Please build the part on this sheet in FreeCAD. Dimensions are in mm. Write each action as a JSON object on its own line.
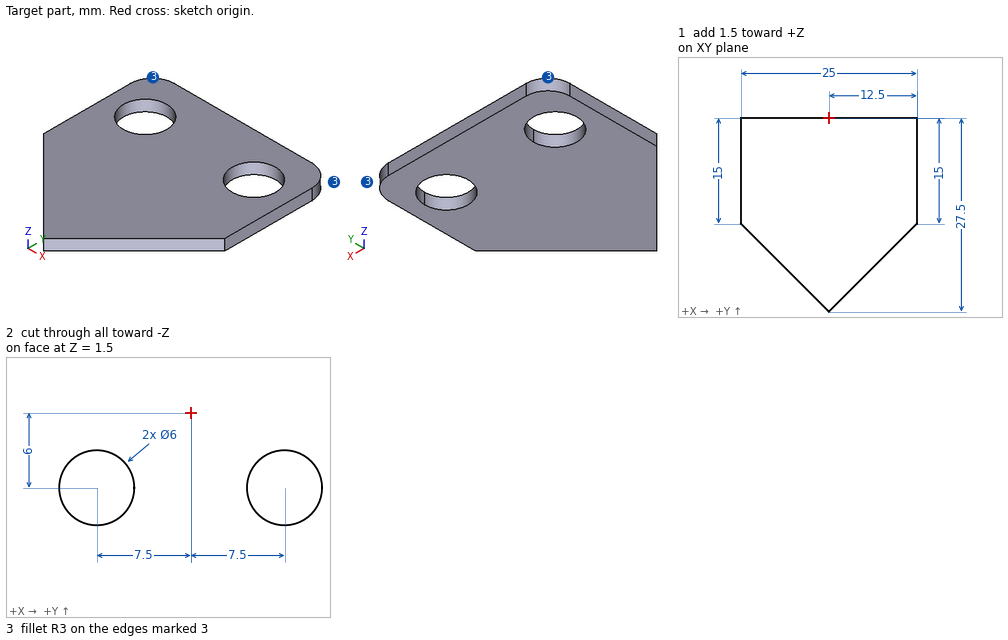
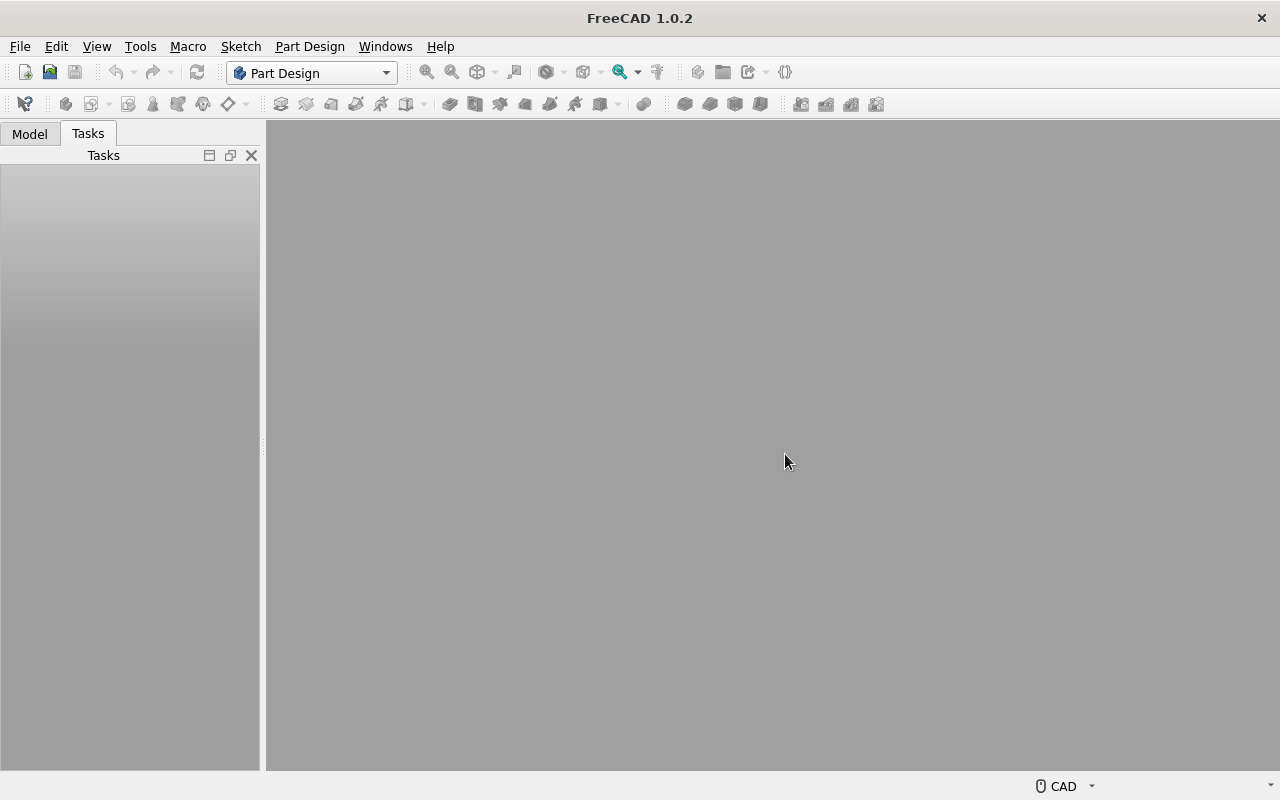
{"action": "left_click", "coordinate": [25, 72]}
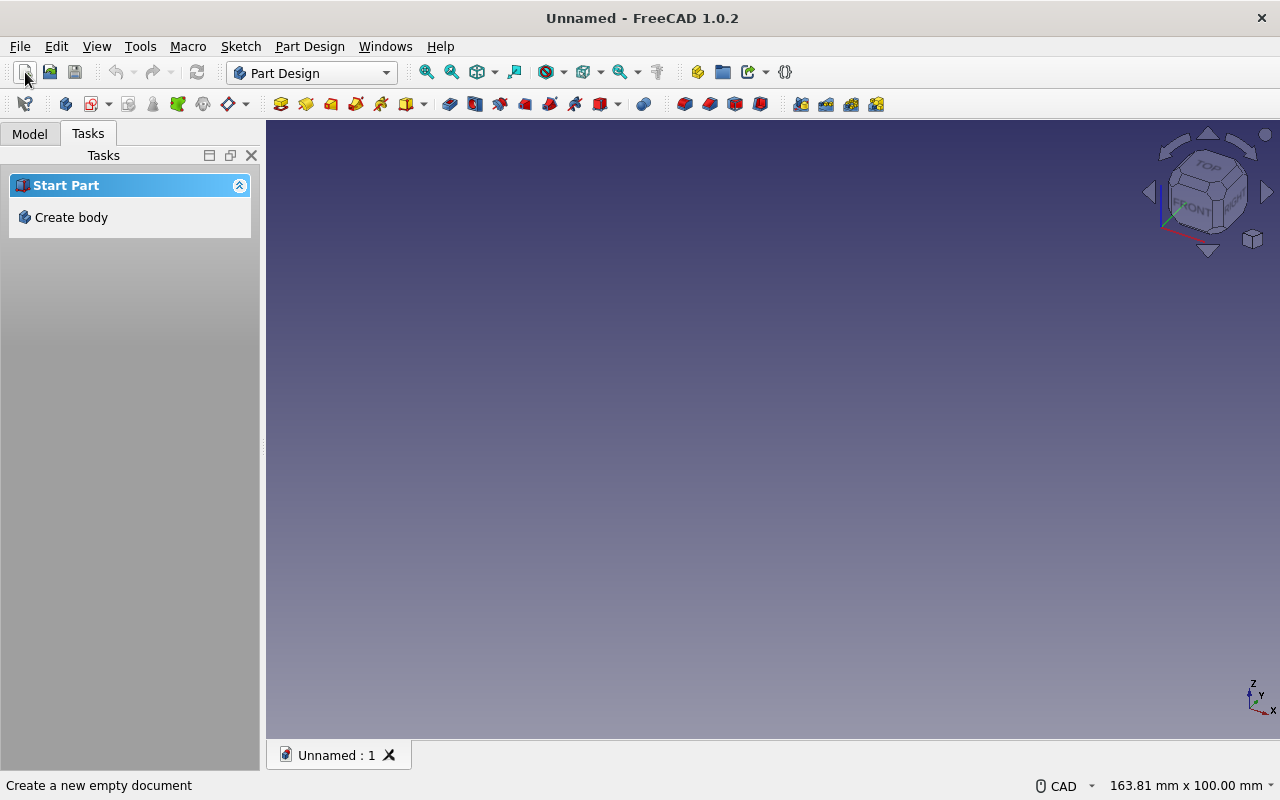
{"action": "left_click", "coordinate": [90, 104]}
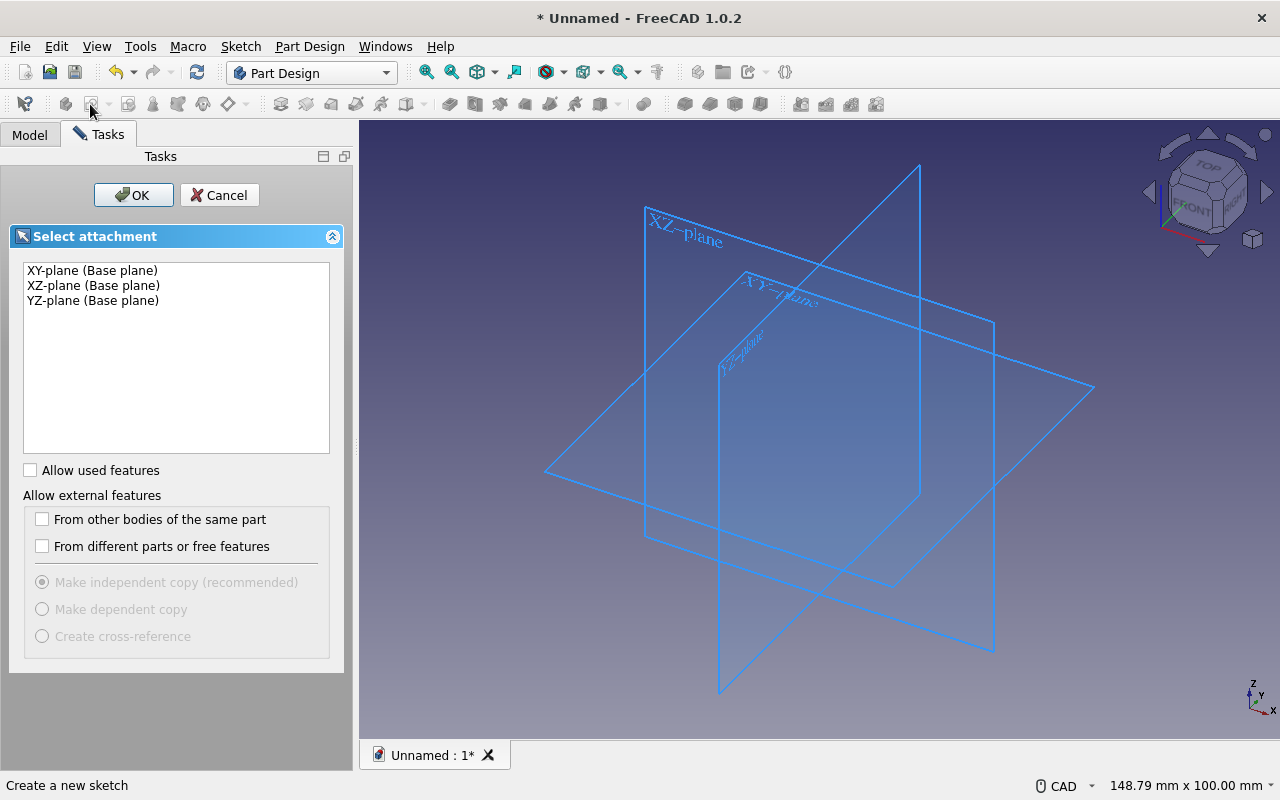
{"action": "left_click", "coordinate": [84, 270]}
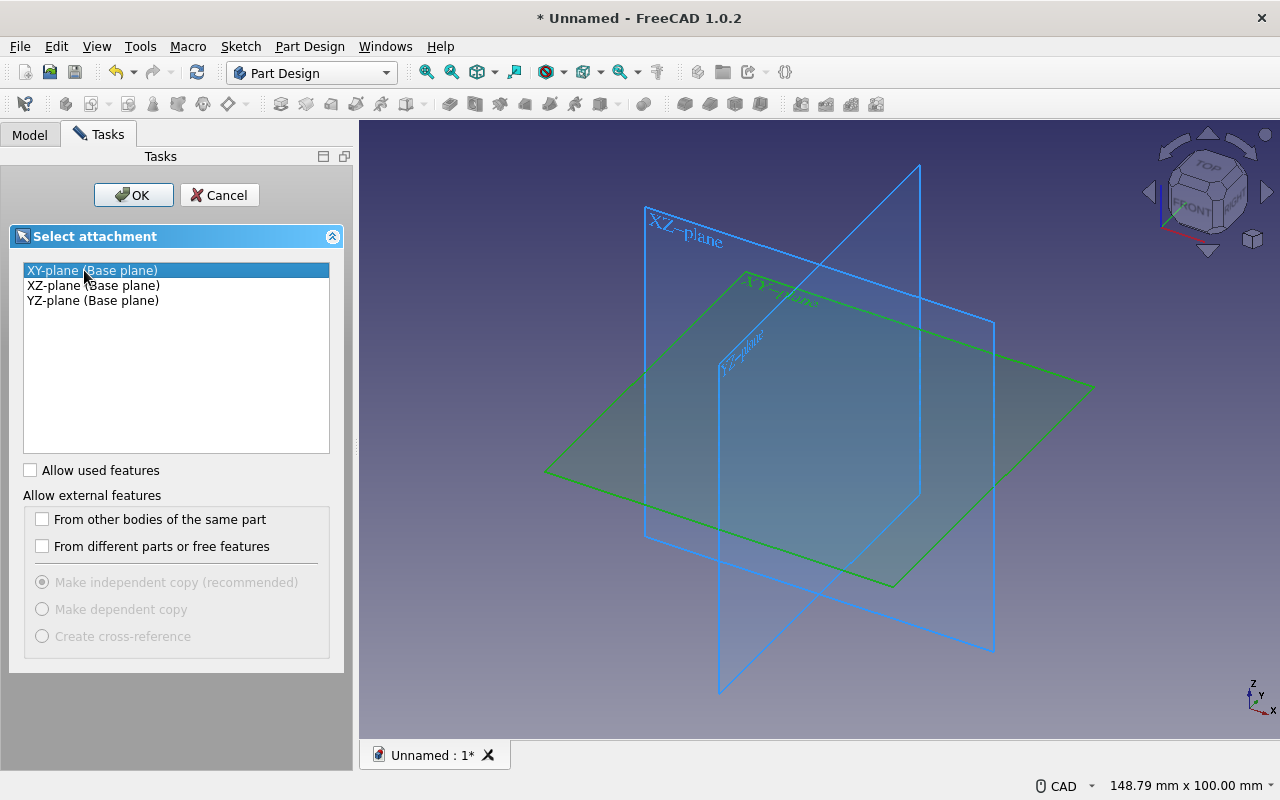
{"action": "left_click", "coordinate": [134, 195]}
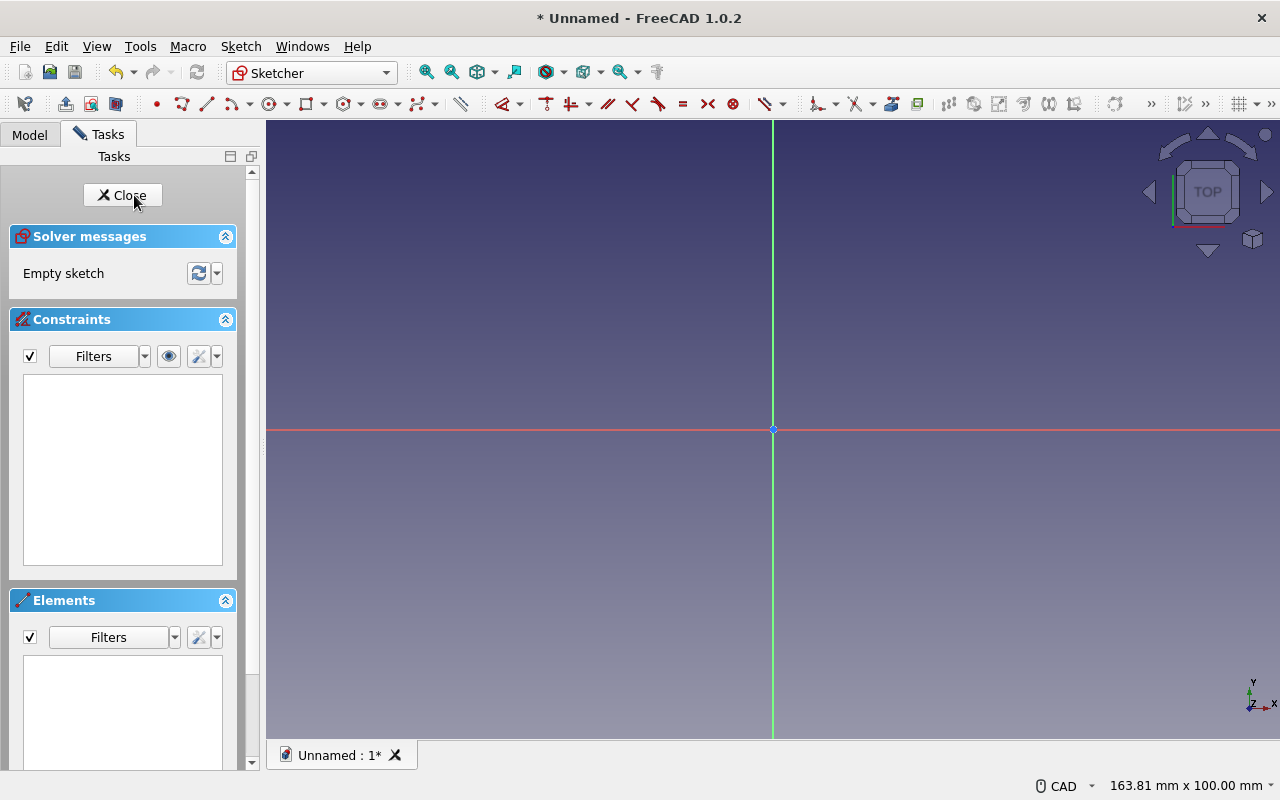
{"action": "scroll", "coordinate": [829, 584], "scroll_direction": "up", "scroll_amount": 4}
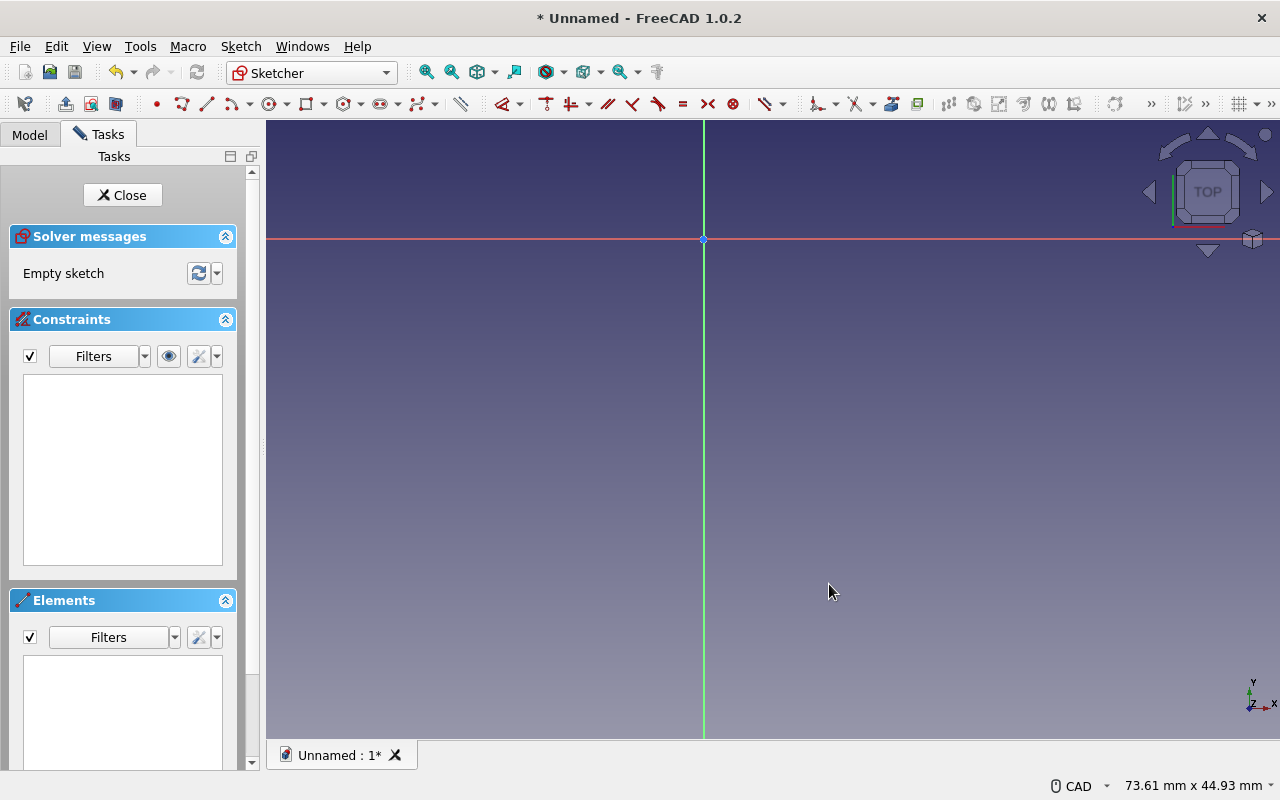
{"action": "left_click", "coordinate": [182, 104]}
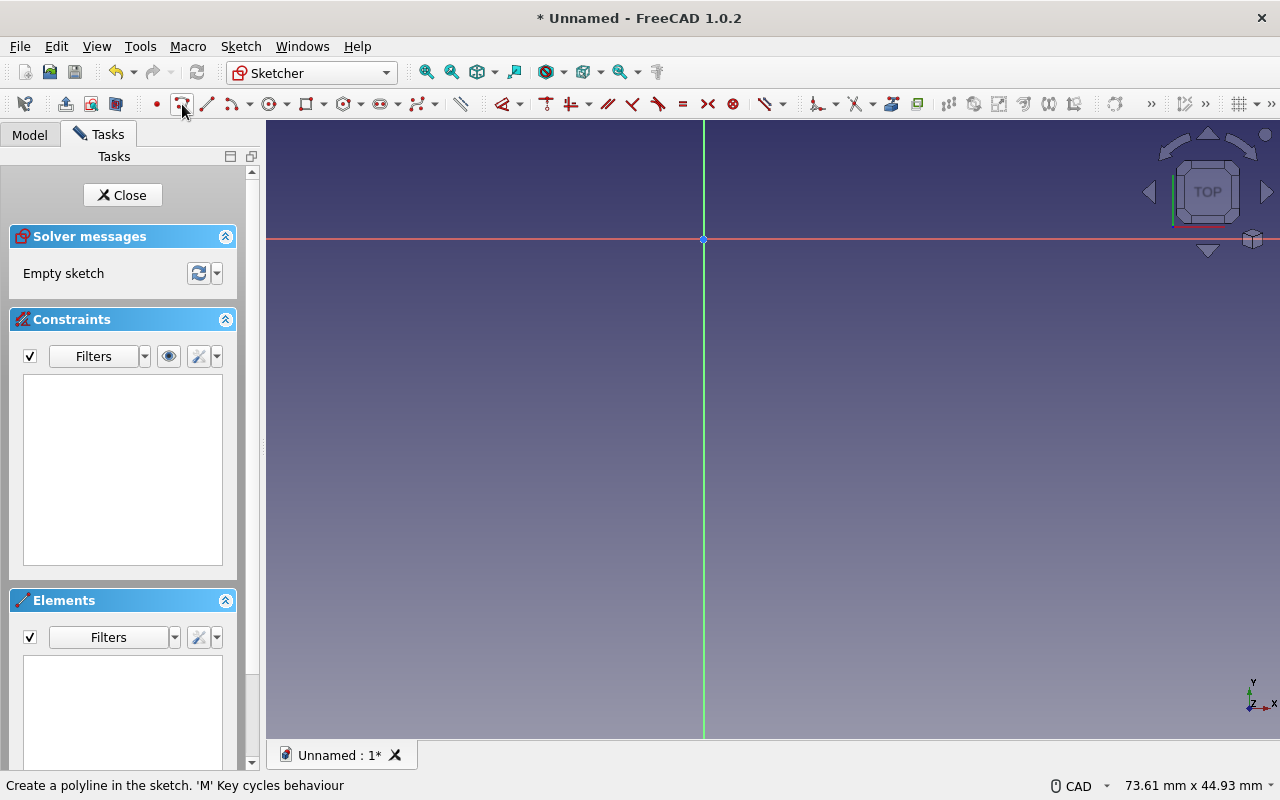
{"action": "left_click", "coordinate": [876, 239]}
{"action": "left_click", "coordinate": [531, 248]}
{"action": "left_click", "coordinate": [531, 446]}
{"action": "left_click", "coordinate": [704, 618]}
{"action": "left_click", "coordinate": [876, 446]}
{"action": "left_click", "coordinate": [876, 239]}
{"action": "key", "text": "Escape"}
{"action": "key", "text": "Escape"}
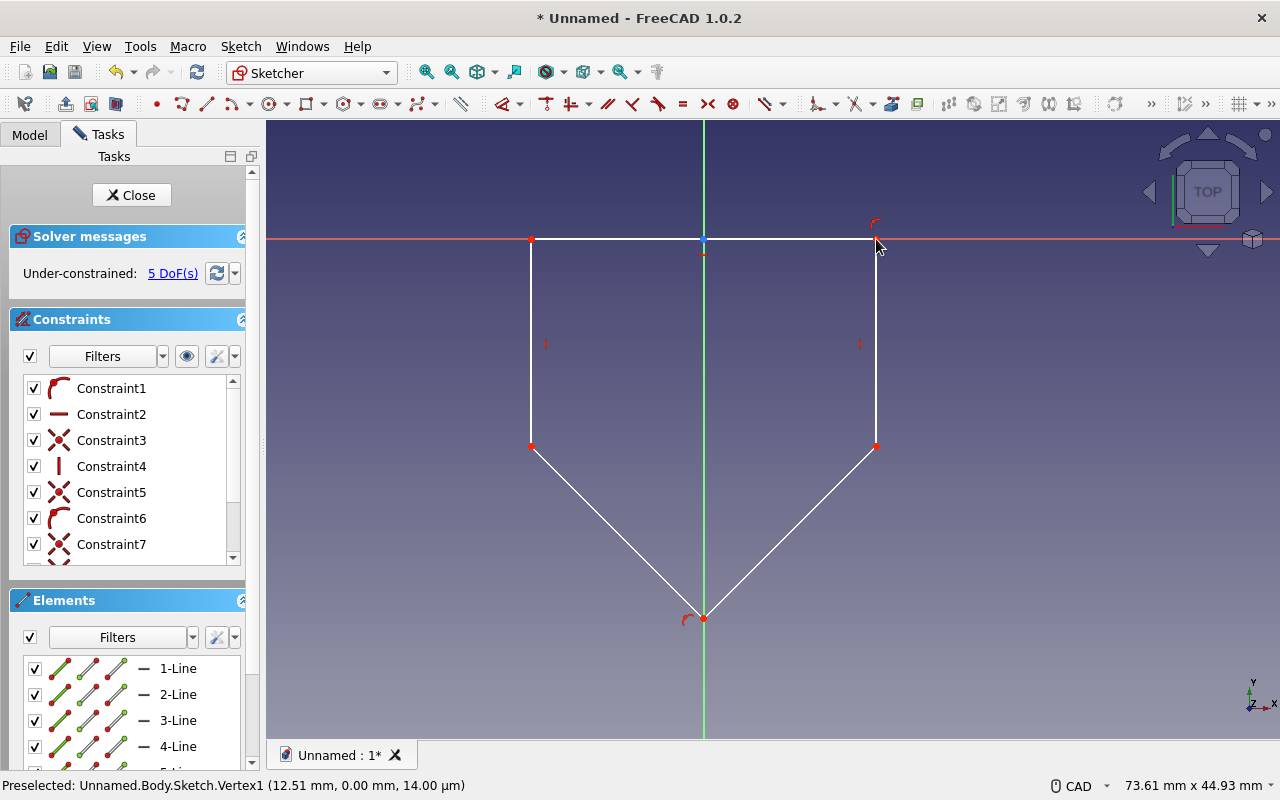
{"action": "left_click", "coordinate": [773, 239]}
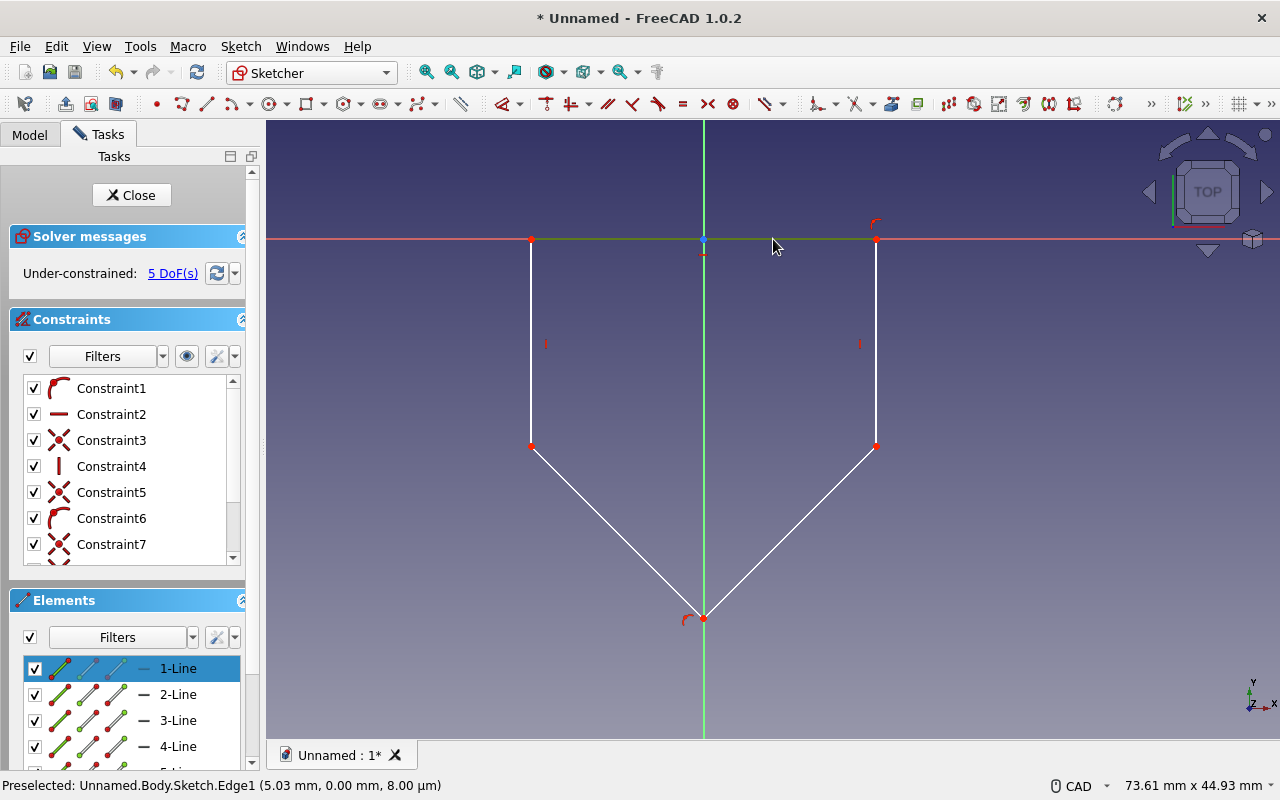
{"action": "key", "text": "l"}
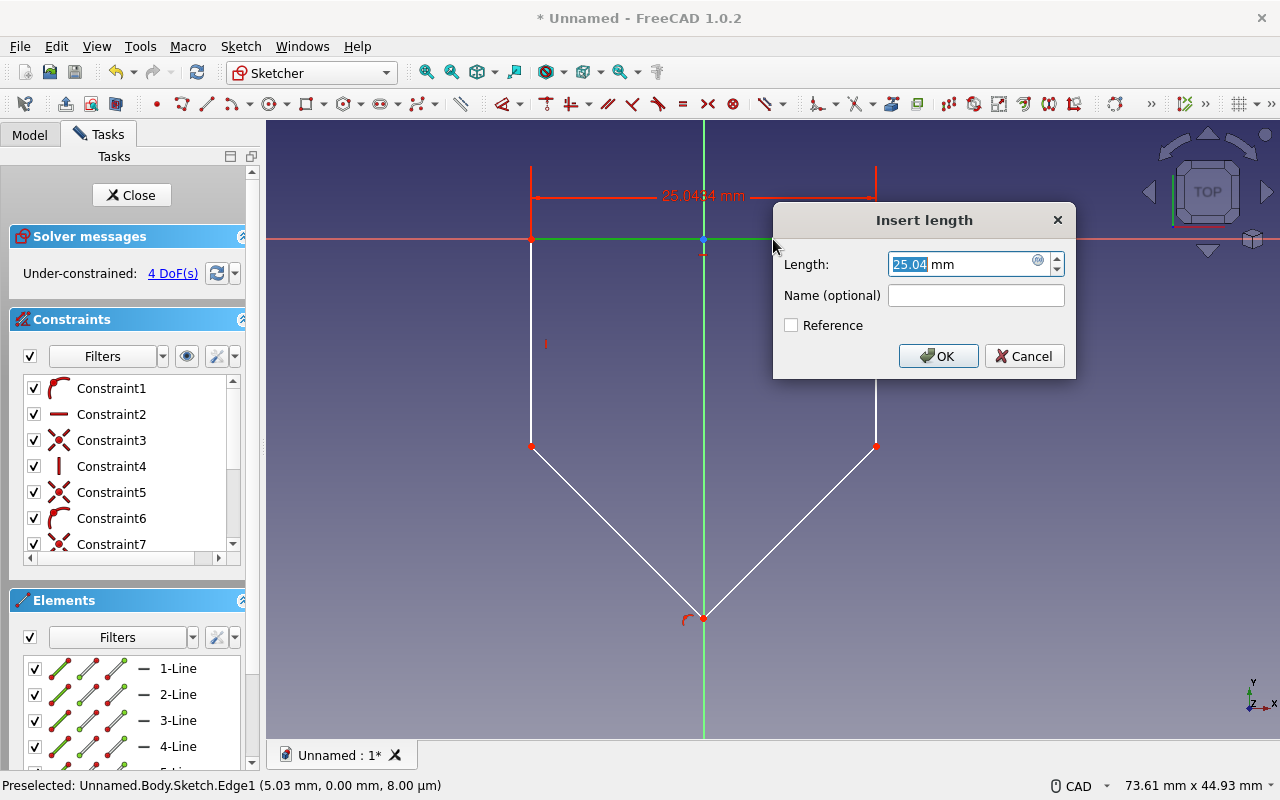
{"action": "type", "text": "25"}
{"action": "key", "text": "Return"}